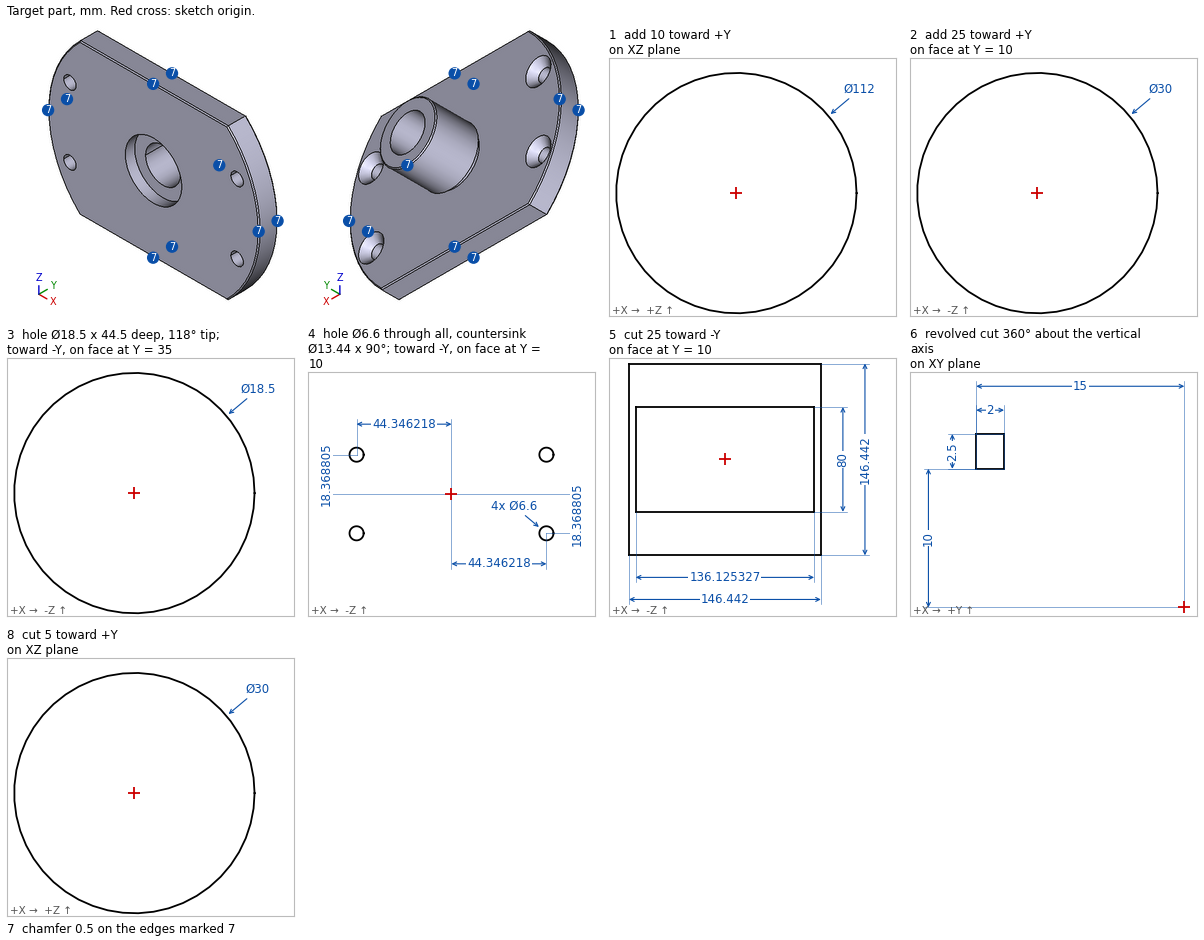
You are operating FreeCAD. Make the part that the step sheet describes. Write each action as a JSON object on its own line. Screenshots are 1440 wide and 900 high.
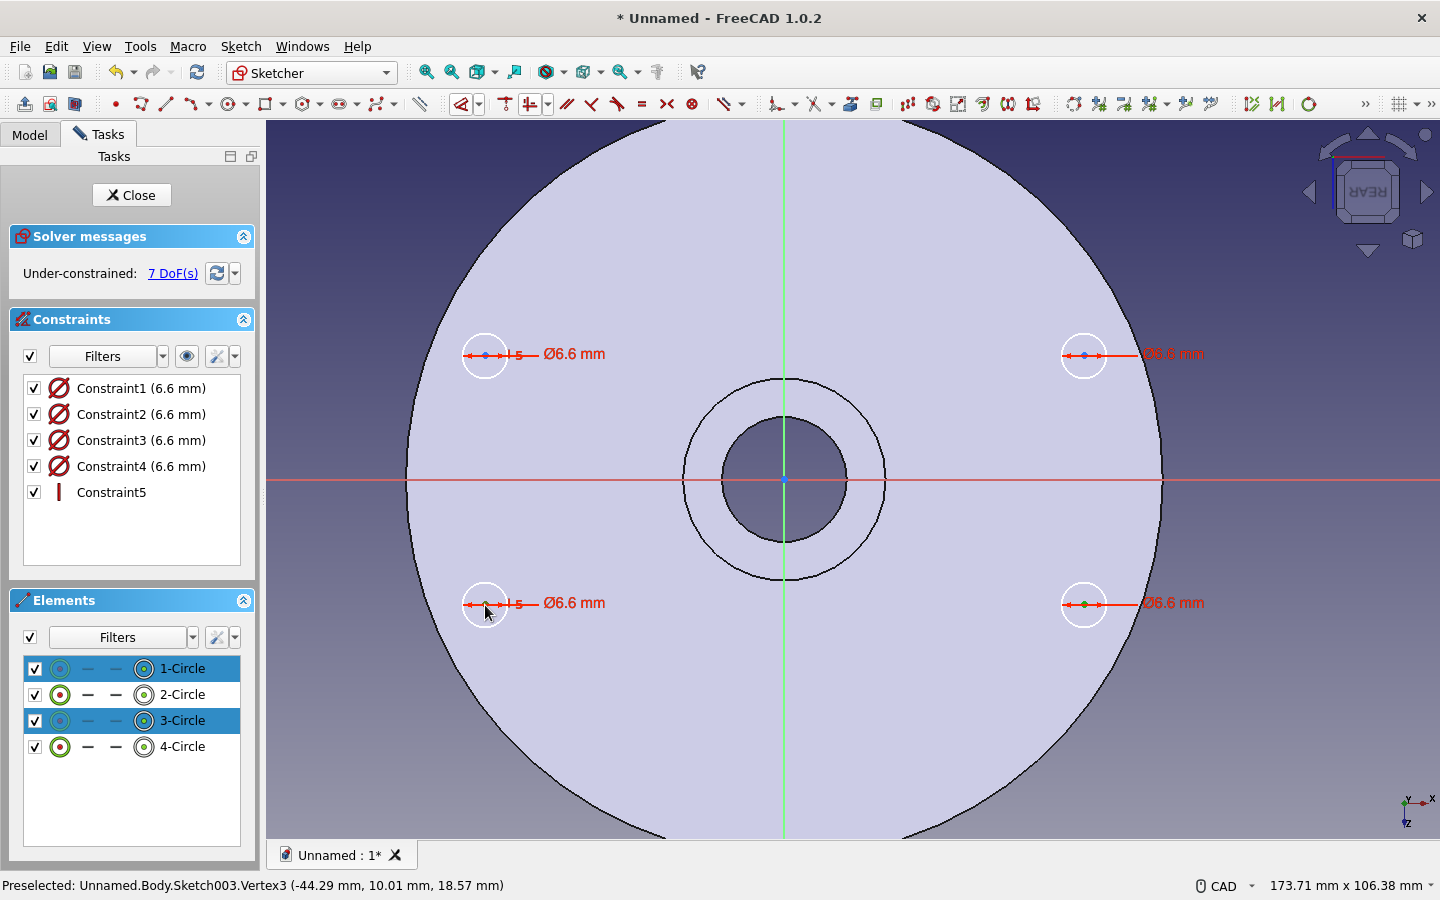
{"action": "left_click", "coordinate": [548, 104]}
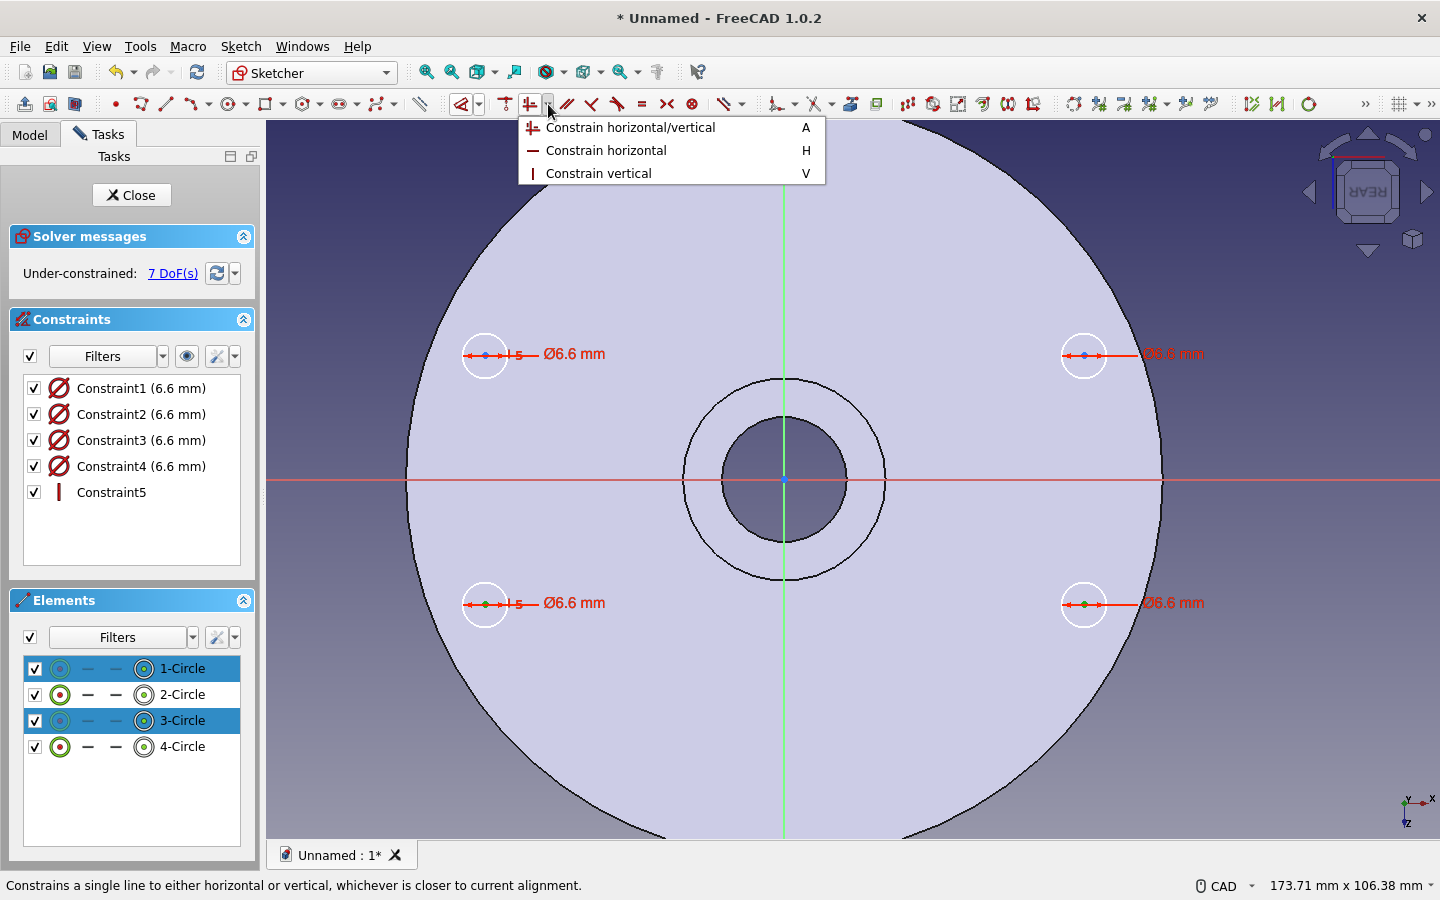
{"action": "left_click", "coordinate": [672, 150]}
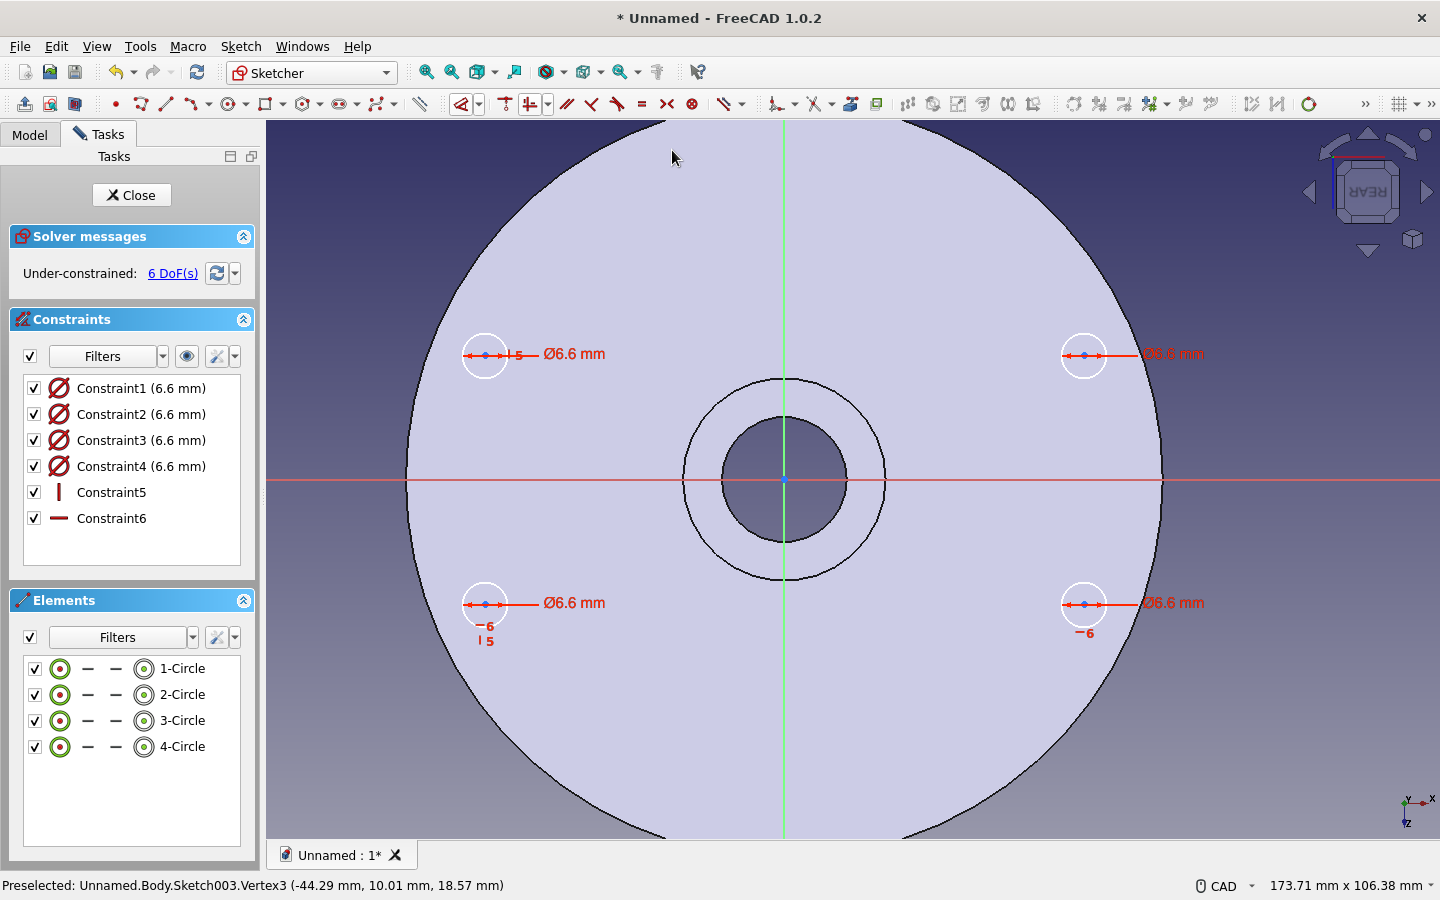
{"action": "left_click", "coordinate": [1084, 605]}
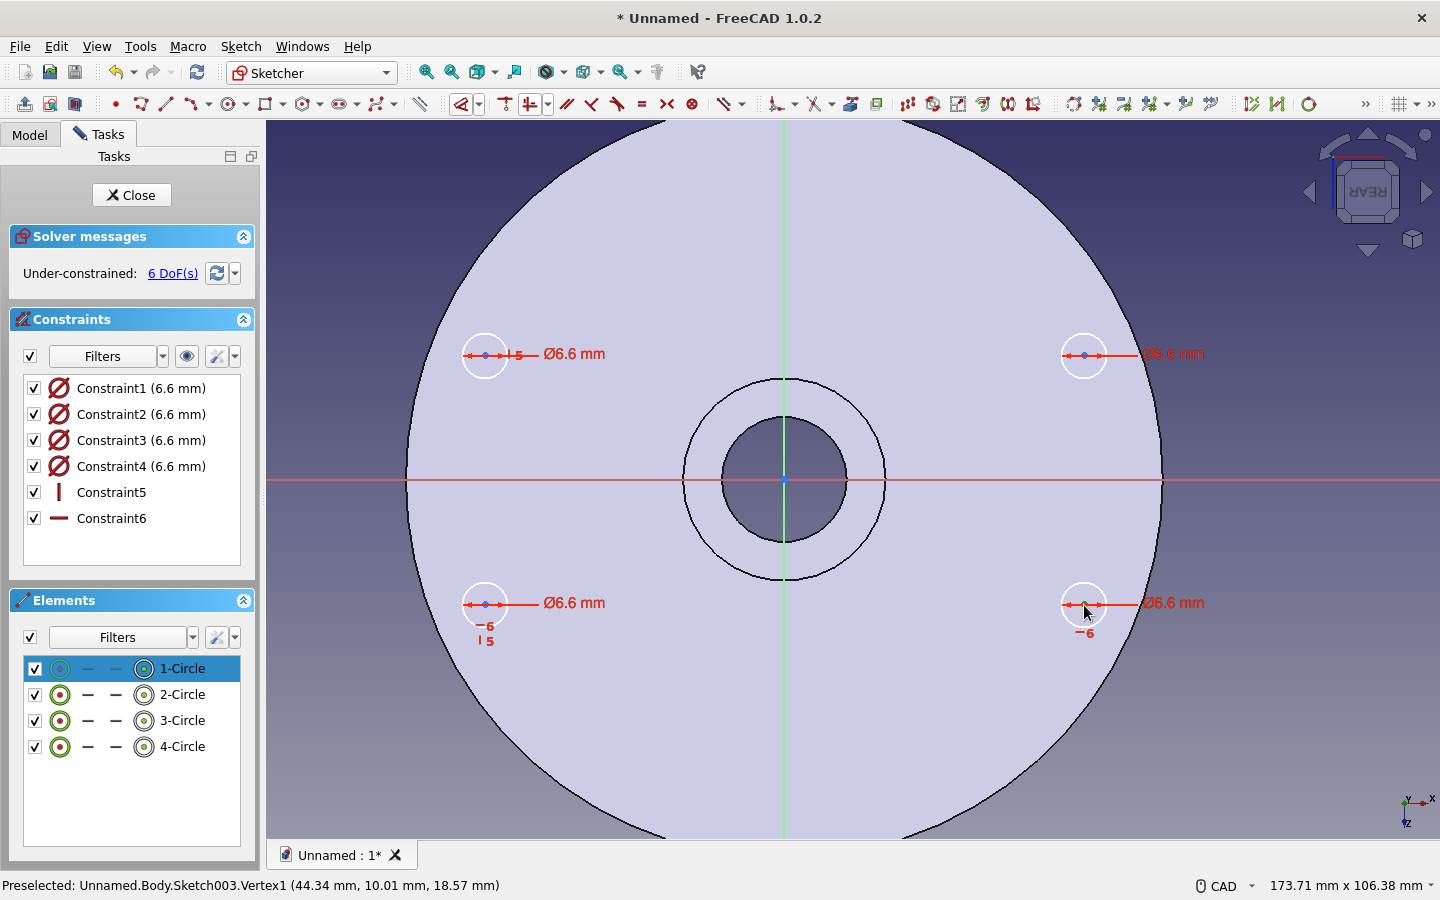
{"action": "left_click", "coordinate": [1084, 356]}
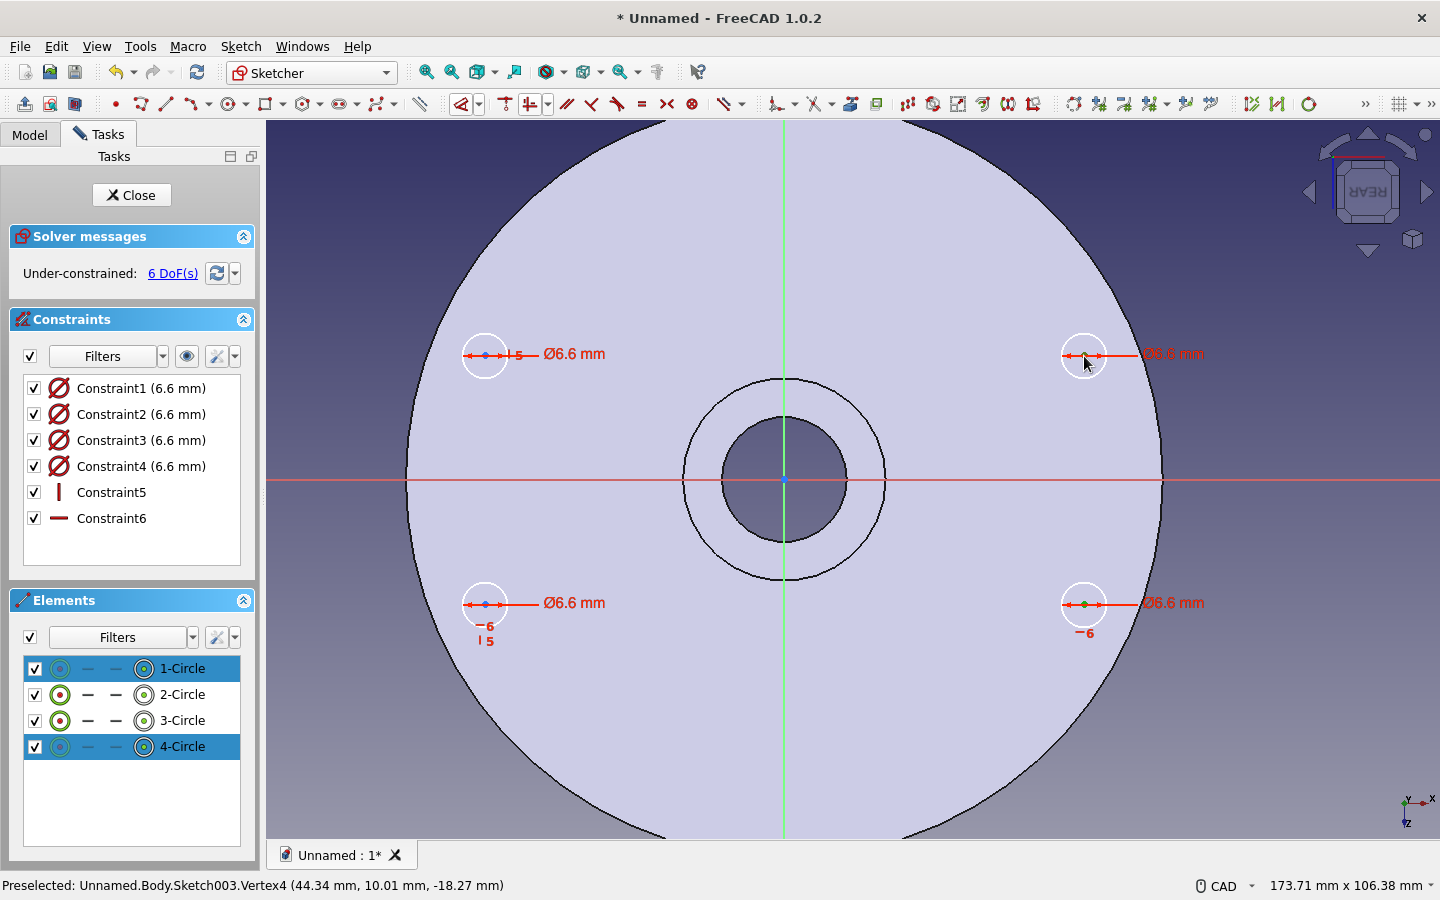
{"action": "key", "text": "v"}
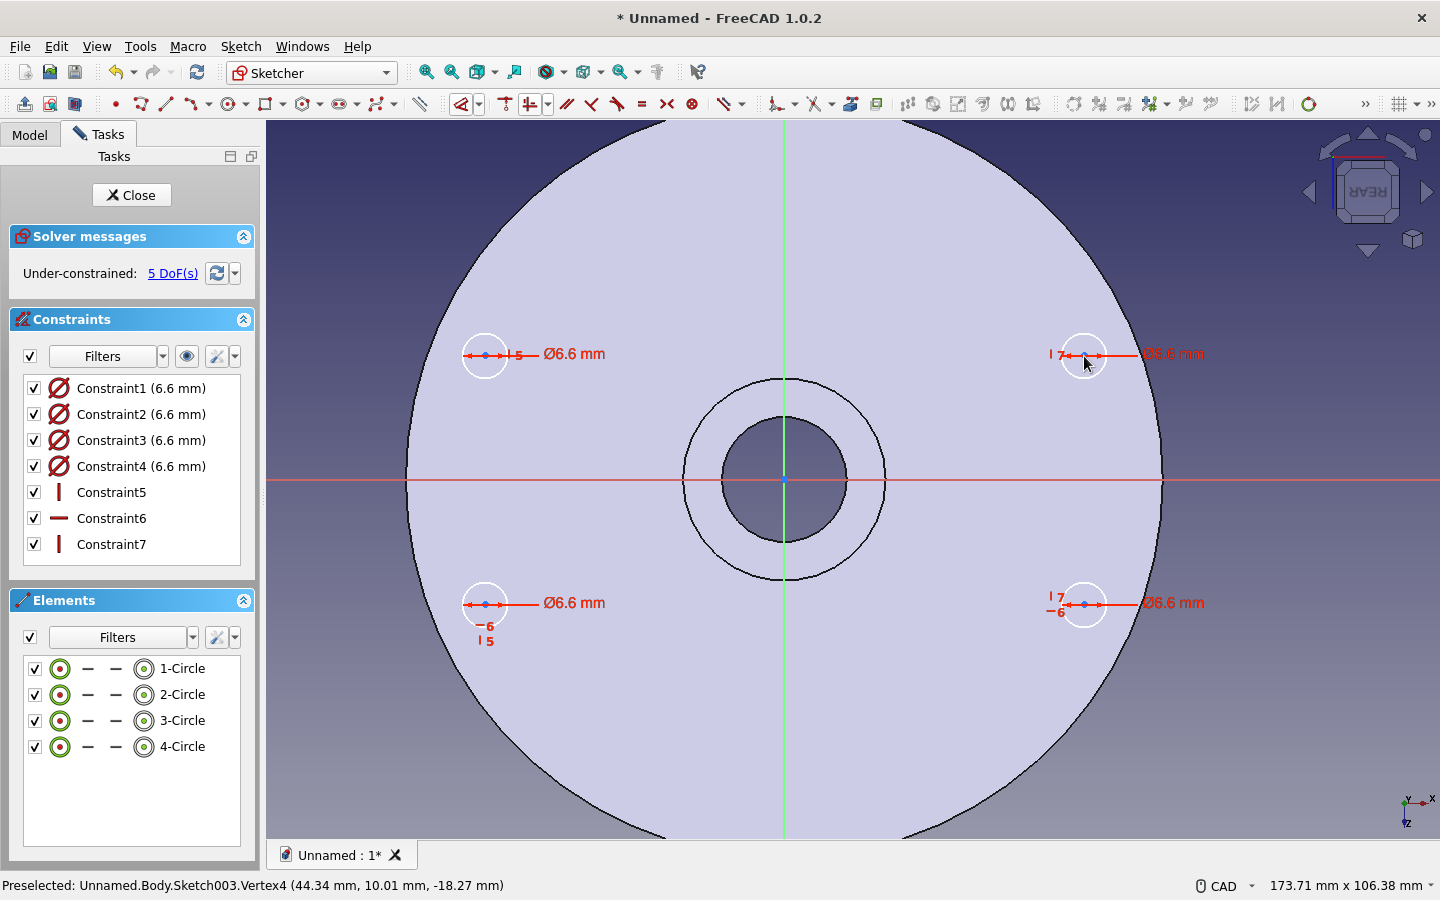
{"action": "left_click", "coordinate": [485, 356]}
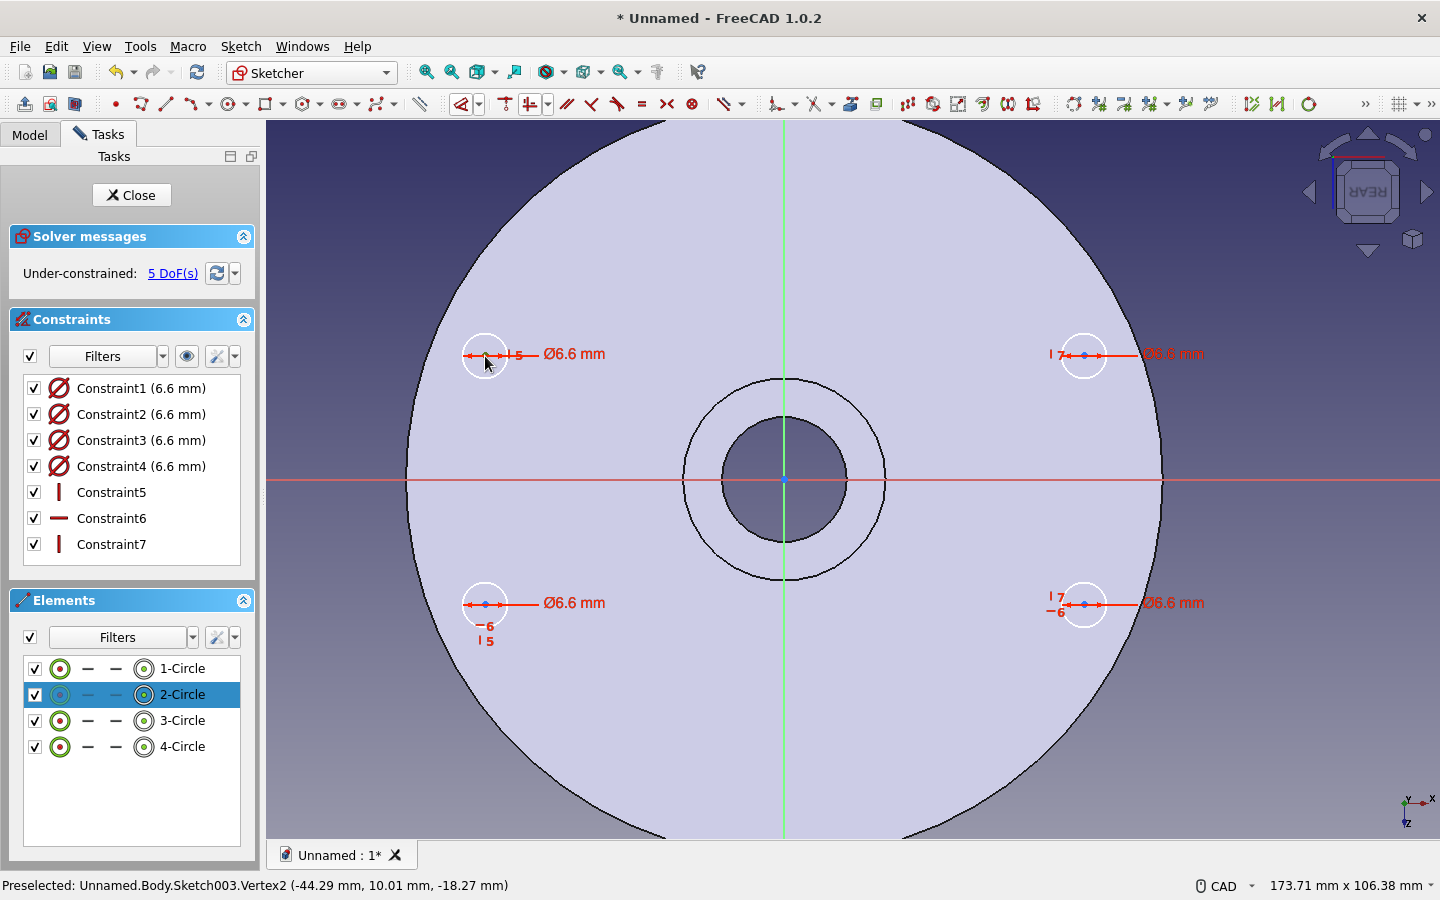
{"action": "left_click", "coordinate": [1084, 356]}